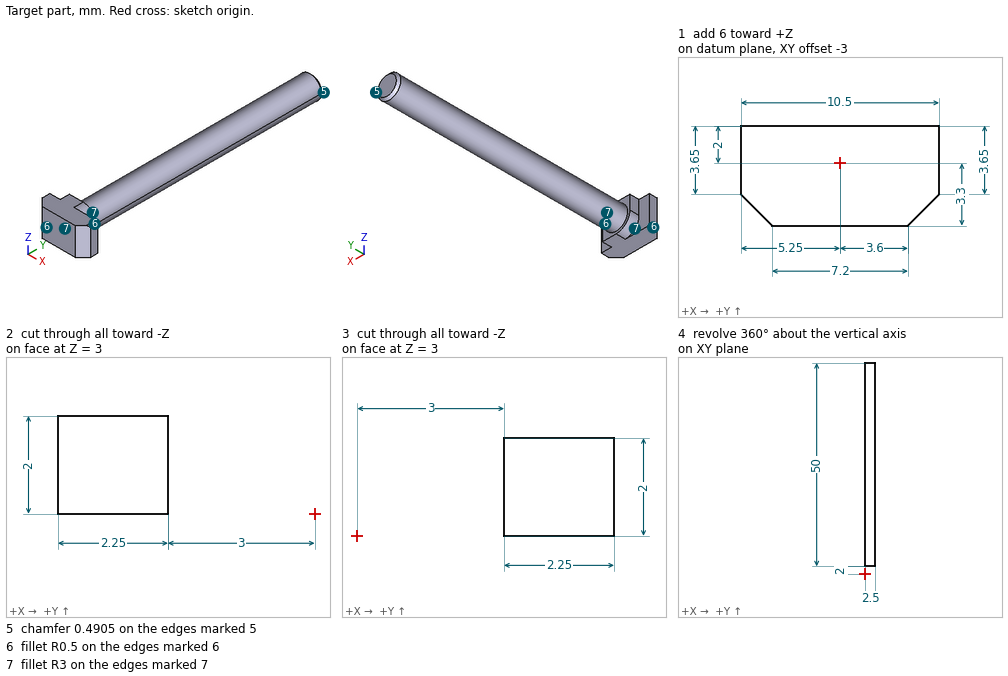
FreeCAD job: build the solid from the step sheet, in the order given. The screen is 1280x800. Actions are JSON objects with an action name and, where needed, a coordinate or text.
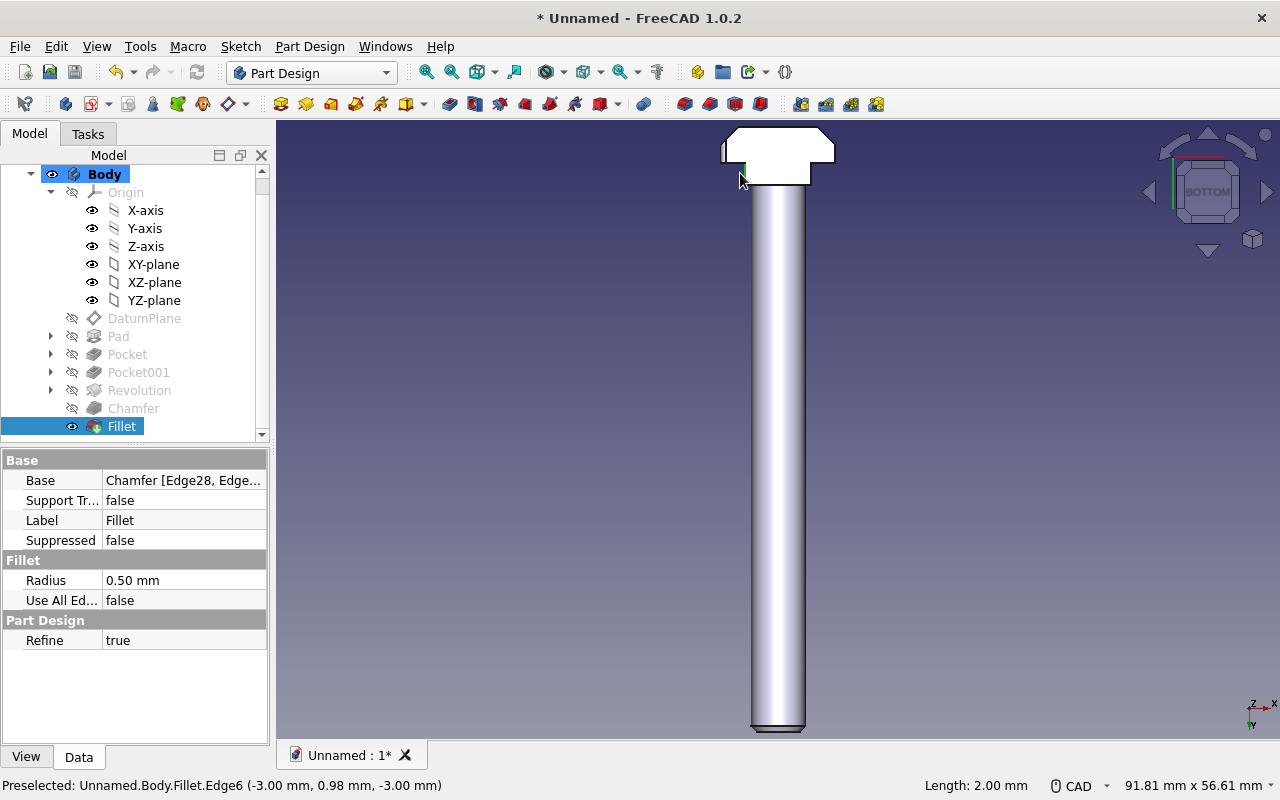
{"action": "scroll", "coordinate": [811, 173], "scroll_direction": "up", "scroll_amount": 4}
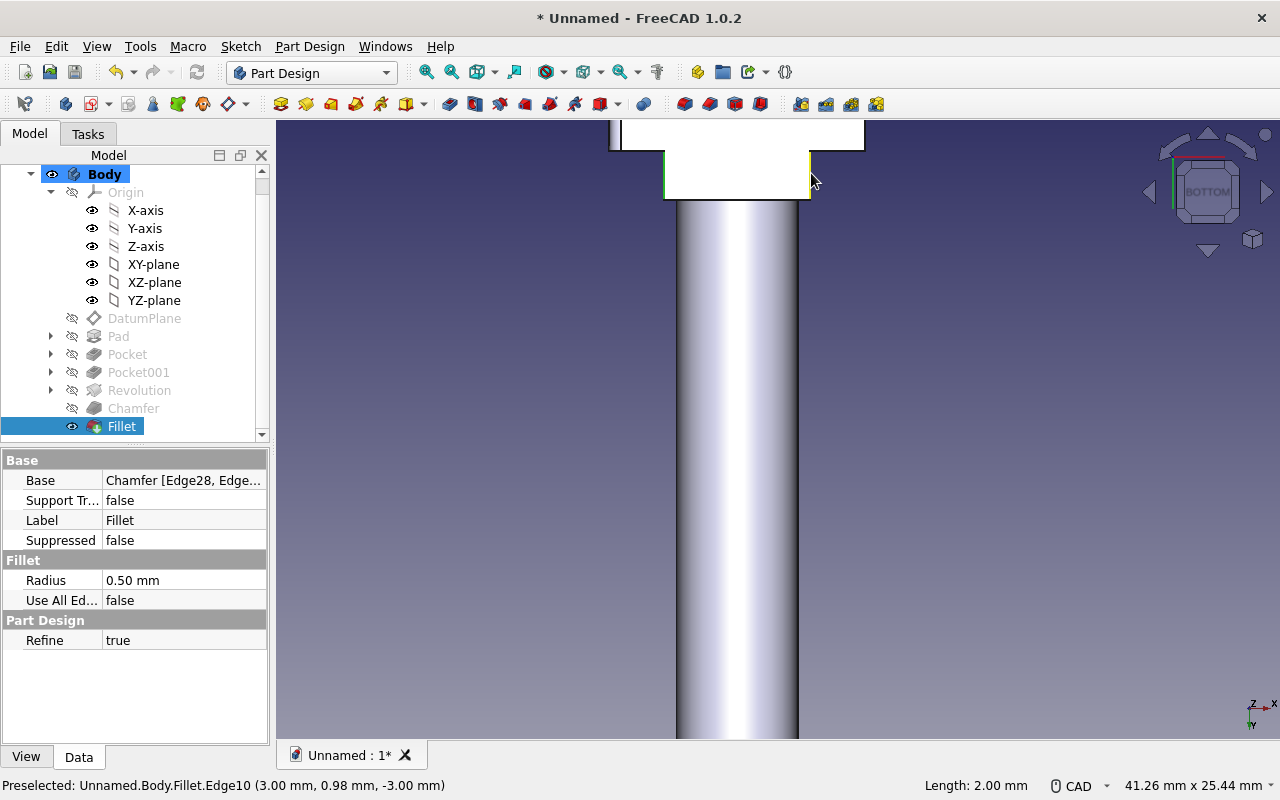
{"action": "key", "text": "v f"}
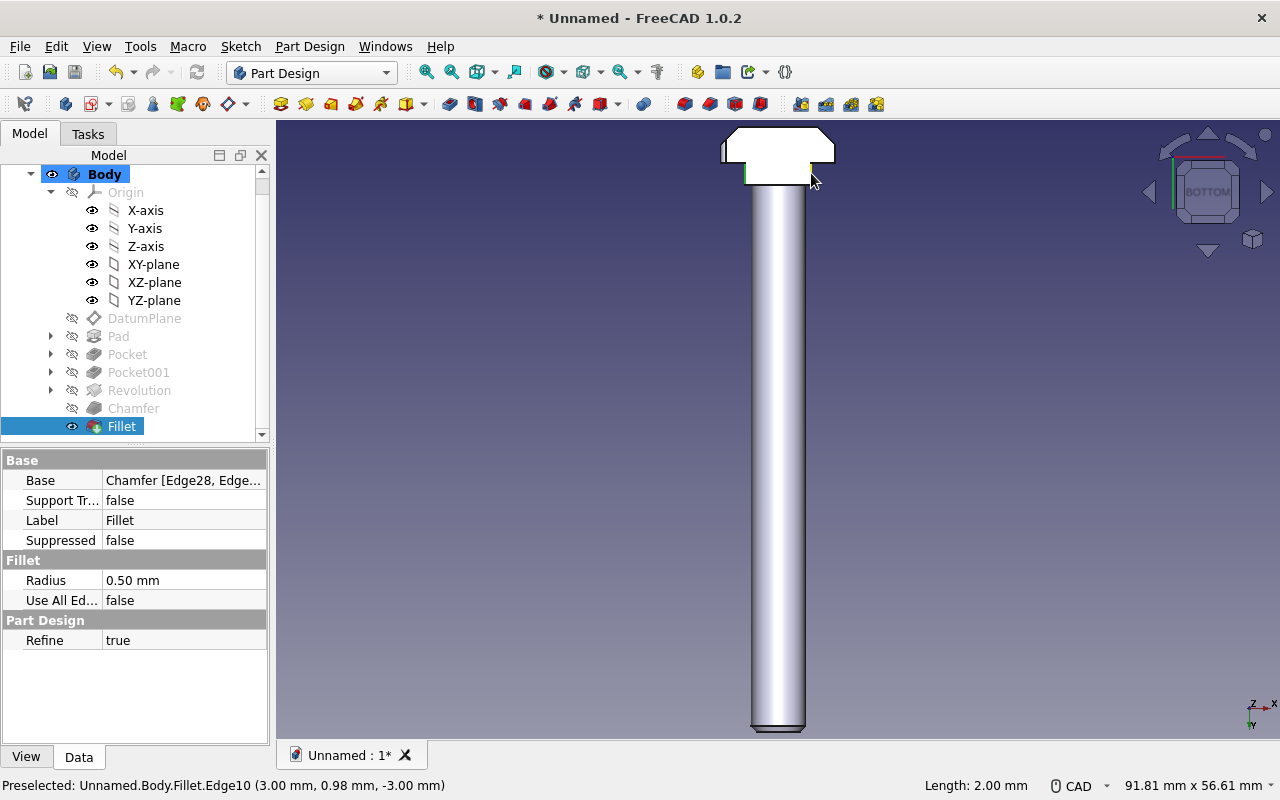
{"action": "key", "text": "0"}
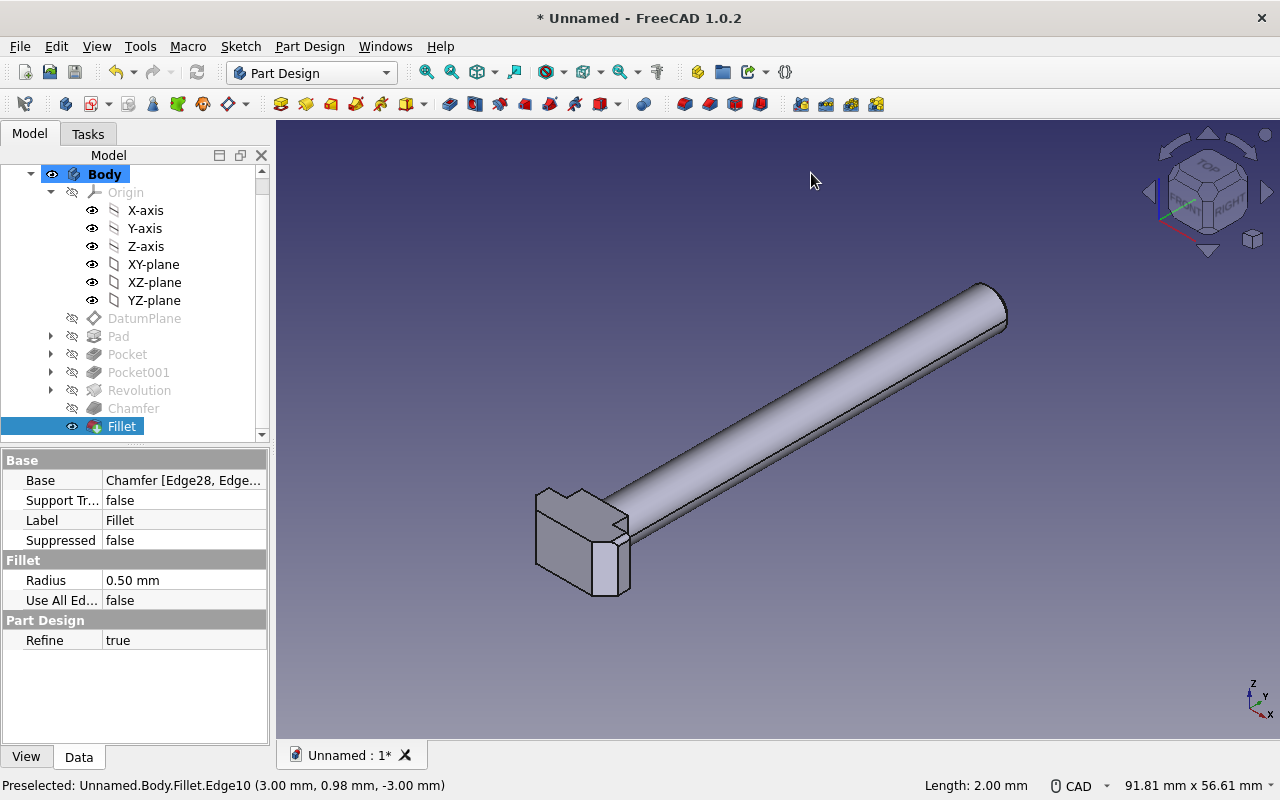
{"action": "left_click", "coordinate": [621, 519], "text": "ctrl"}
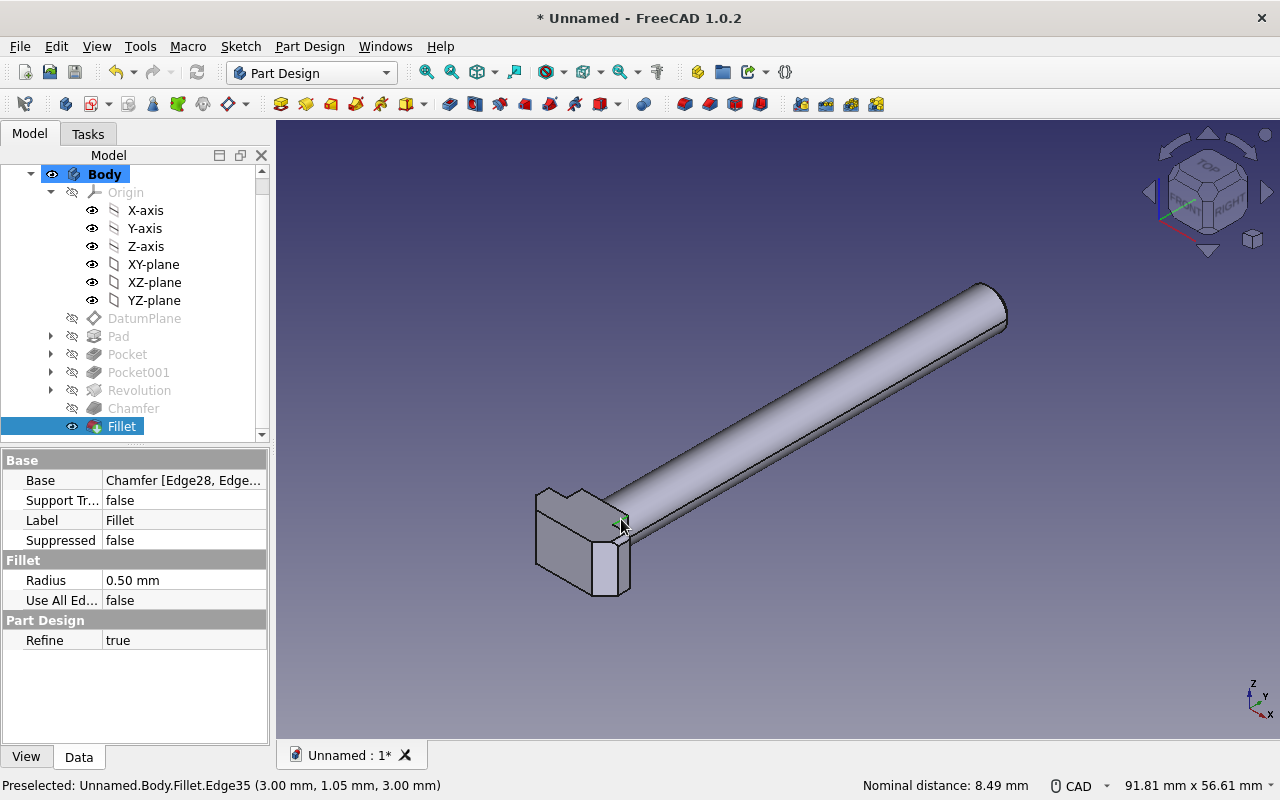
{"action": "left_click", "coordinate": [685, 104]}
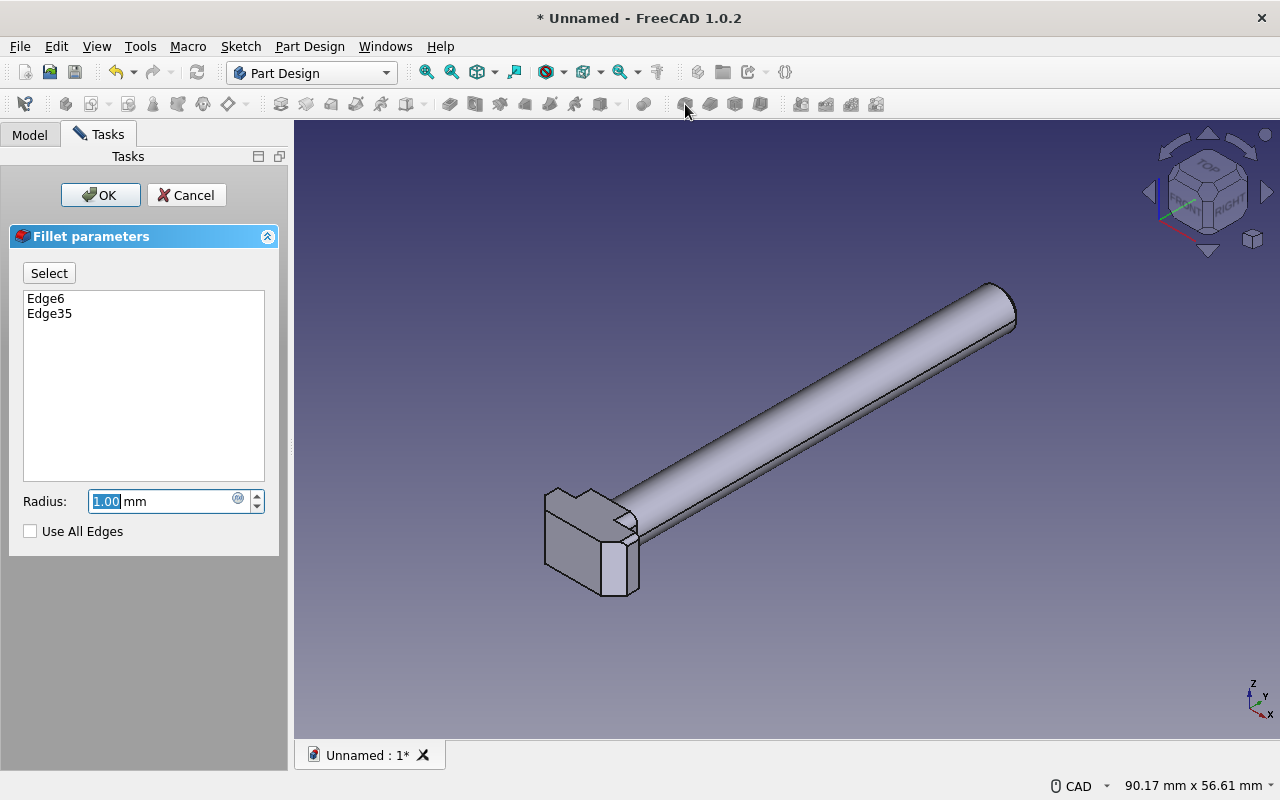
{"action": "type", "text": "3"}
{"action": "key", "text": "Tab"}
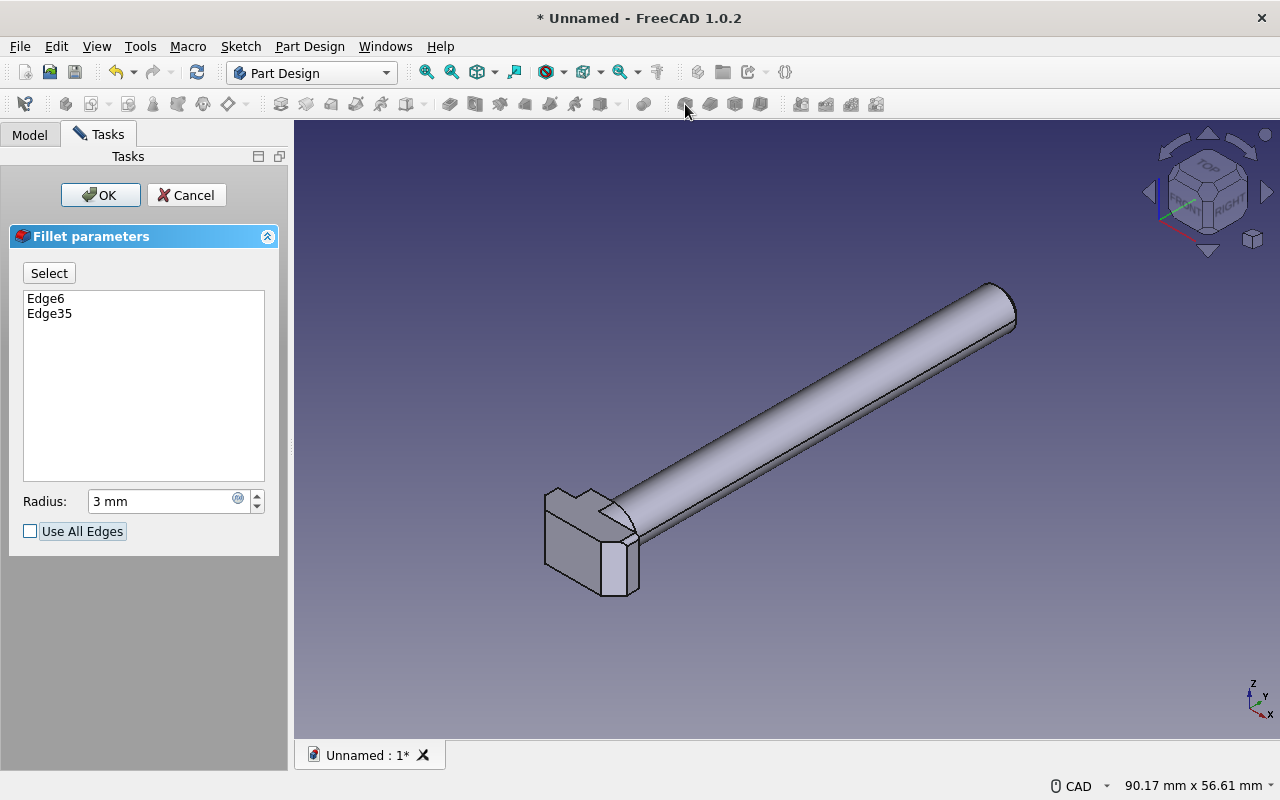
{"action": "left_click", "coordinate": [101, 195]}